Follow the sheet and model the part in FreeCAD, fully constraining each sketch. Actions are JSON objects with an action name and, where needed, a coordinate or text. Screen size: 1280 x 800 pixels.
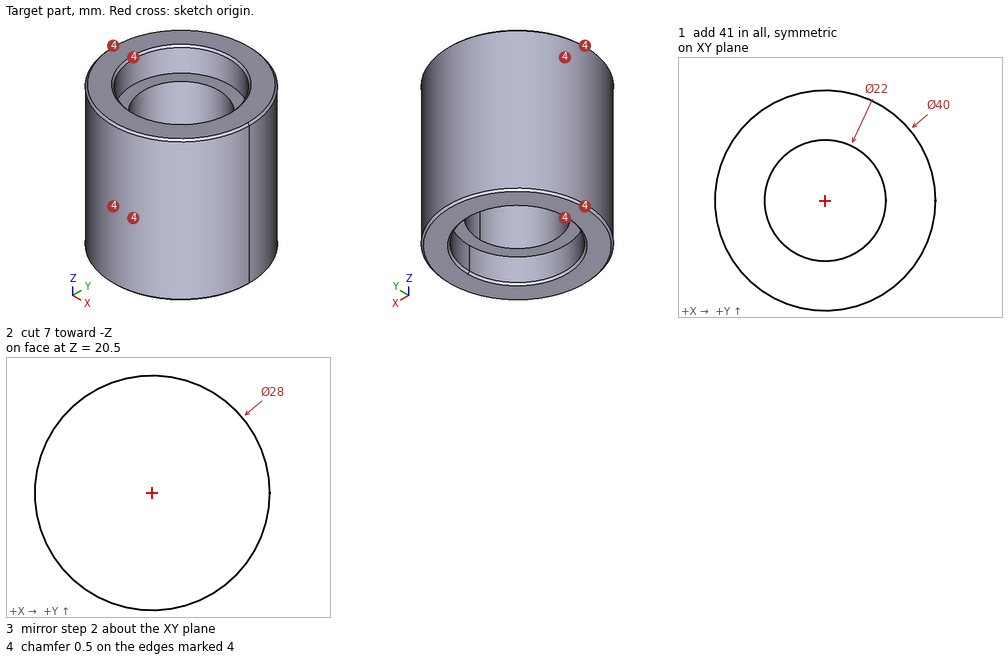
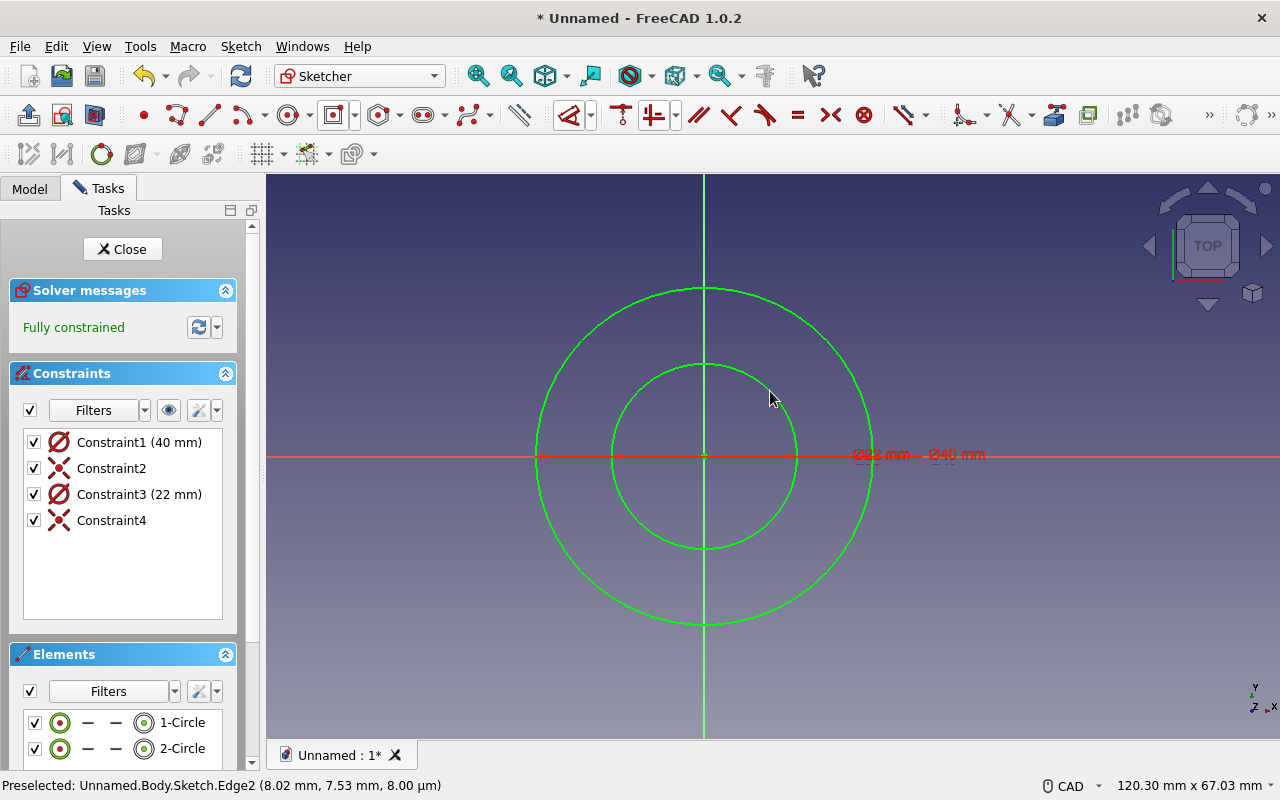
{"action": "left_click", "coordinate": [123, 249]}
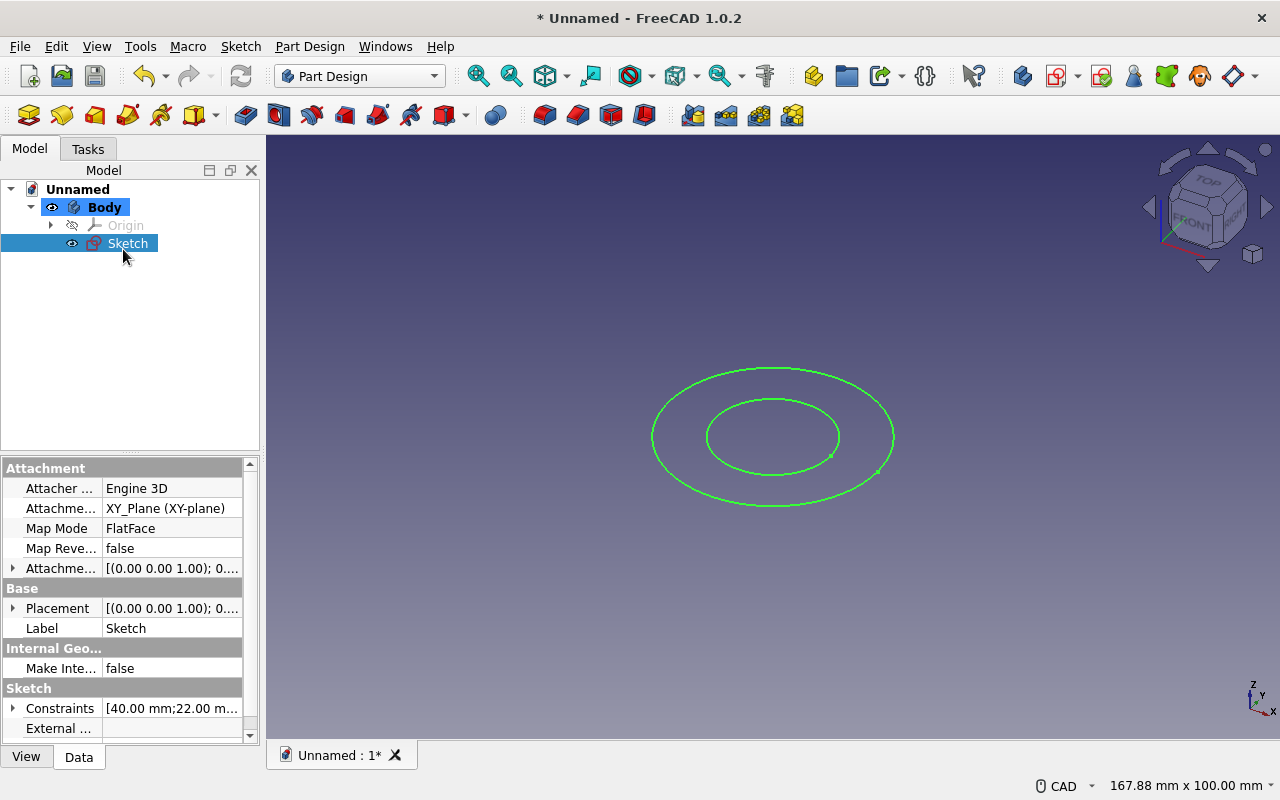
{"action": "left_click", "coordinate": [29, 116]}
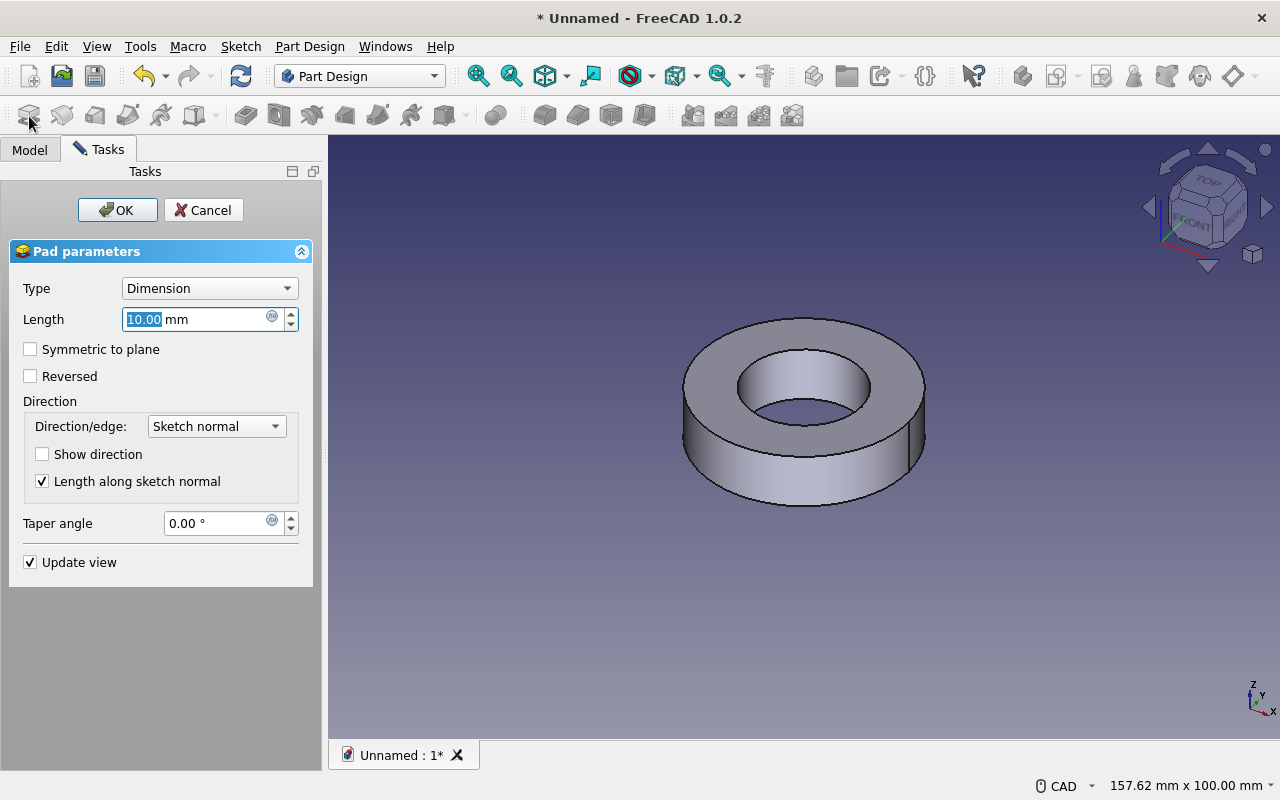
{"action": "type", "text": "41"}
{"action": "key", "text": "Tab"}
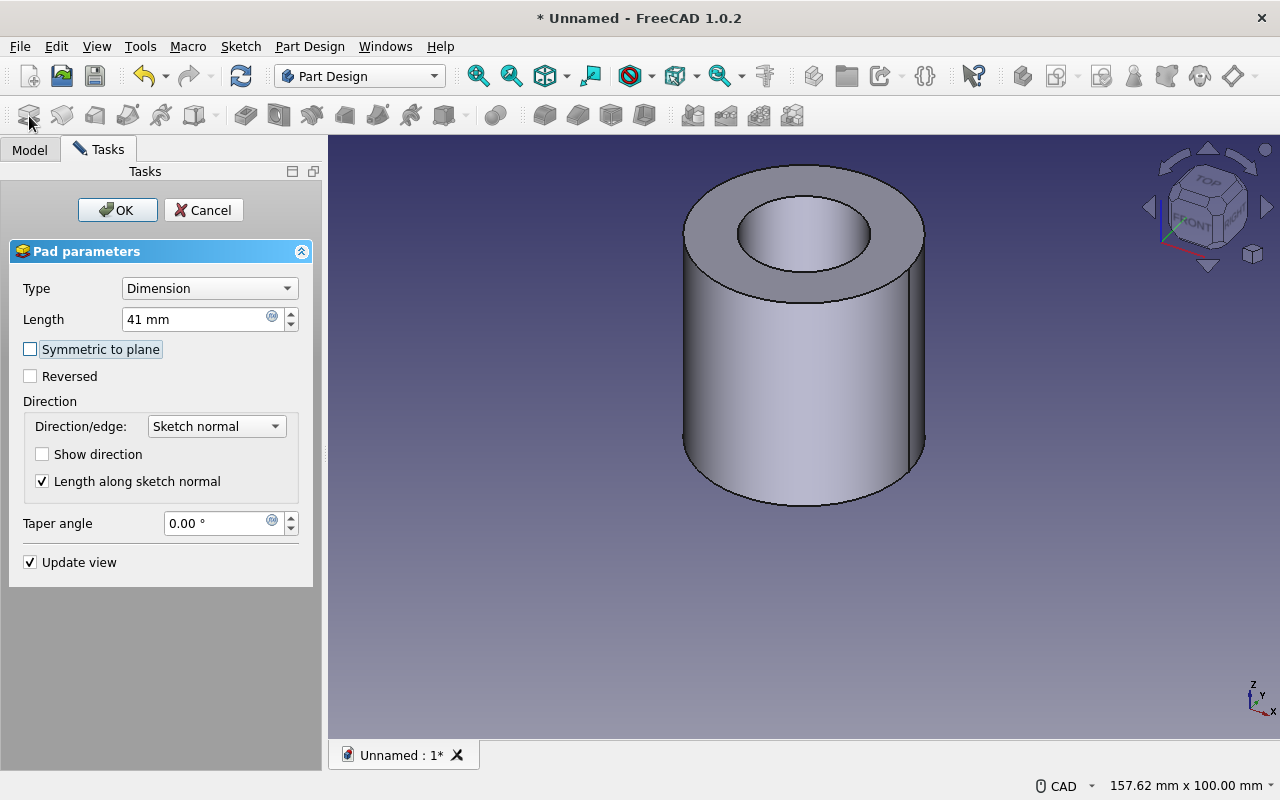
{"action": "left_click", "coordinate": [31, 349]}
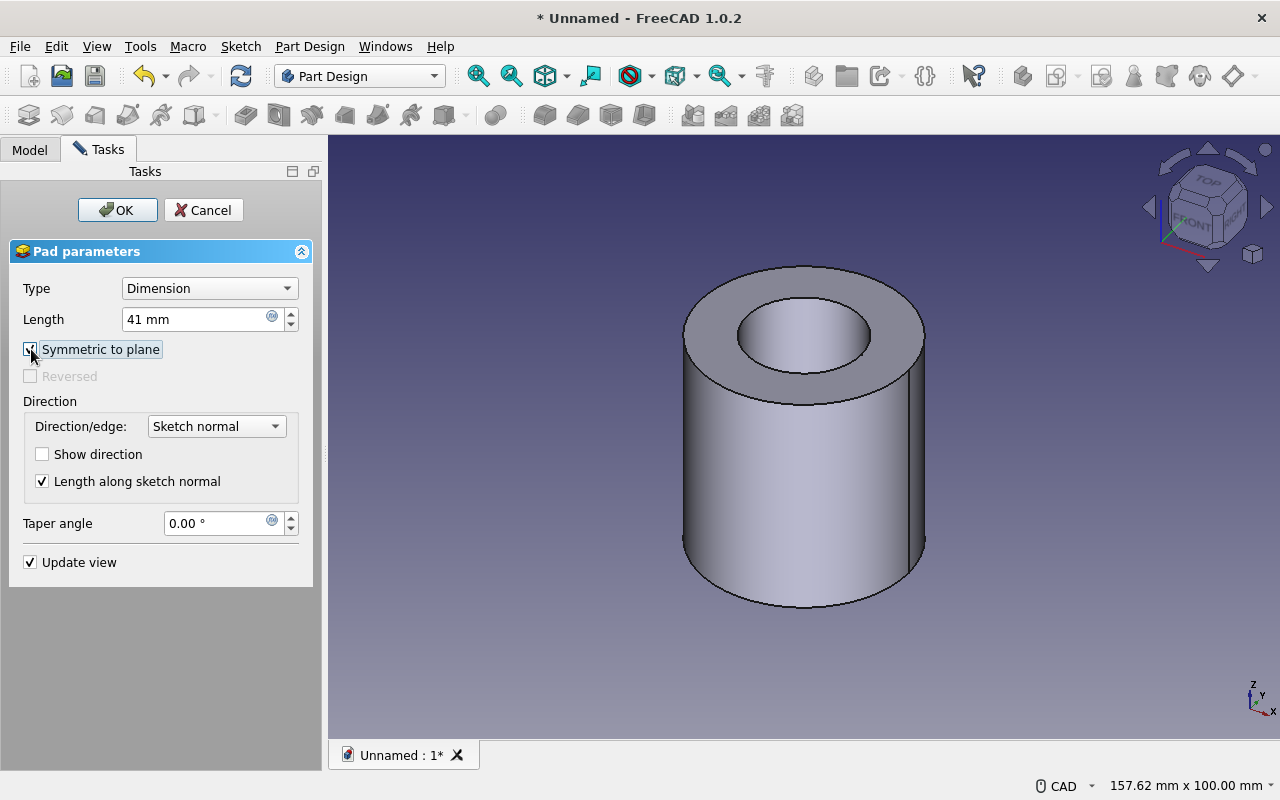
{"action": "left_click", "coordinate": [118, 210]}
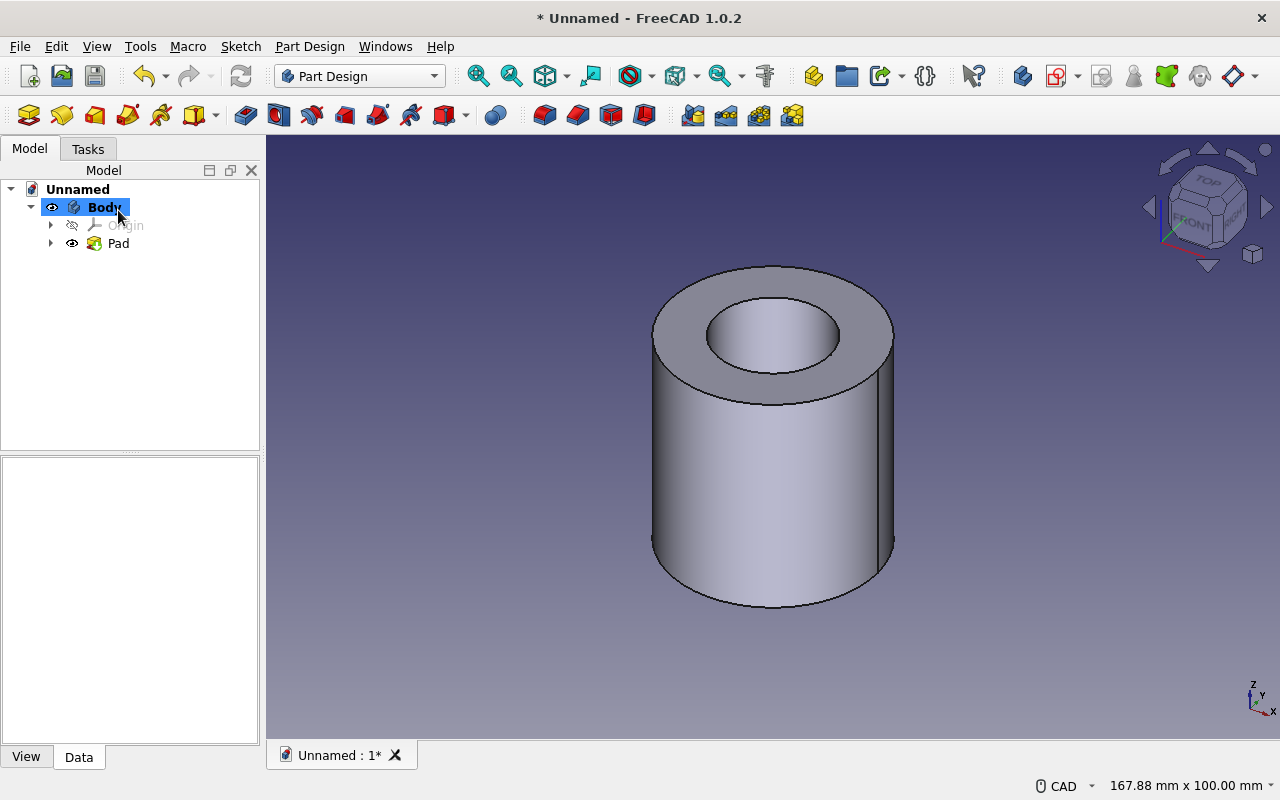
{"action": "left_click", "coordinate": [867, 320]}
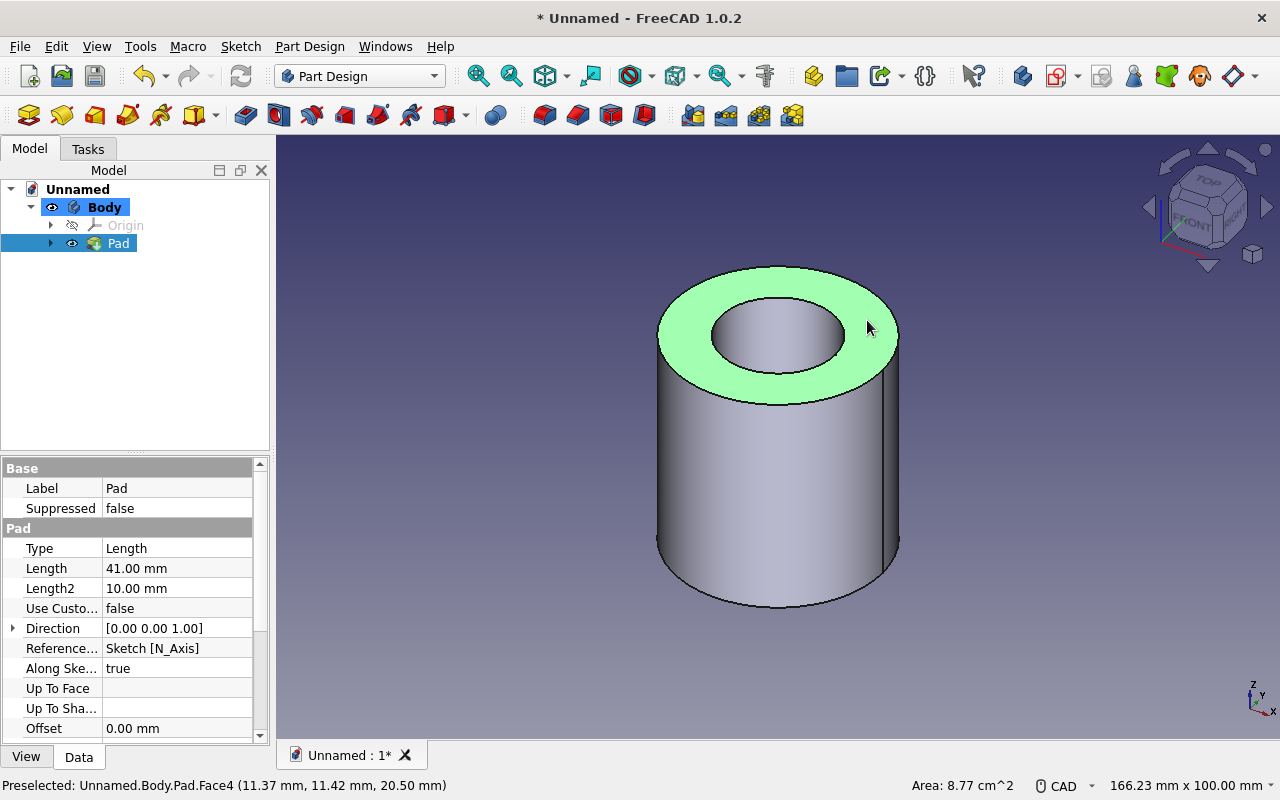
{"action": "left_click", "coordinate": [1056, 76]}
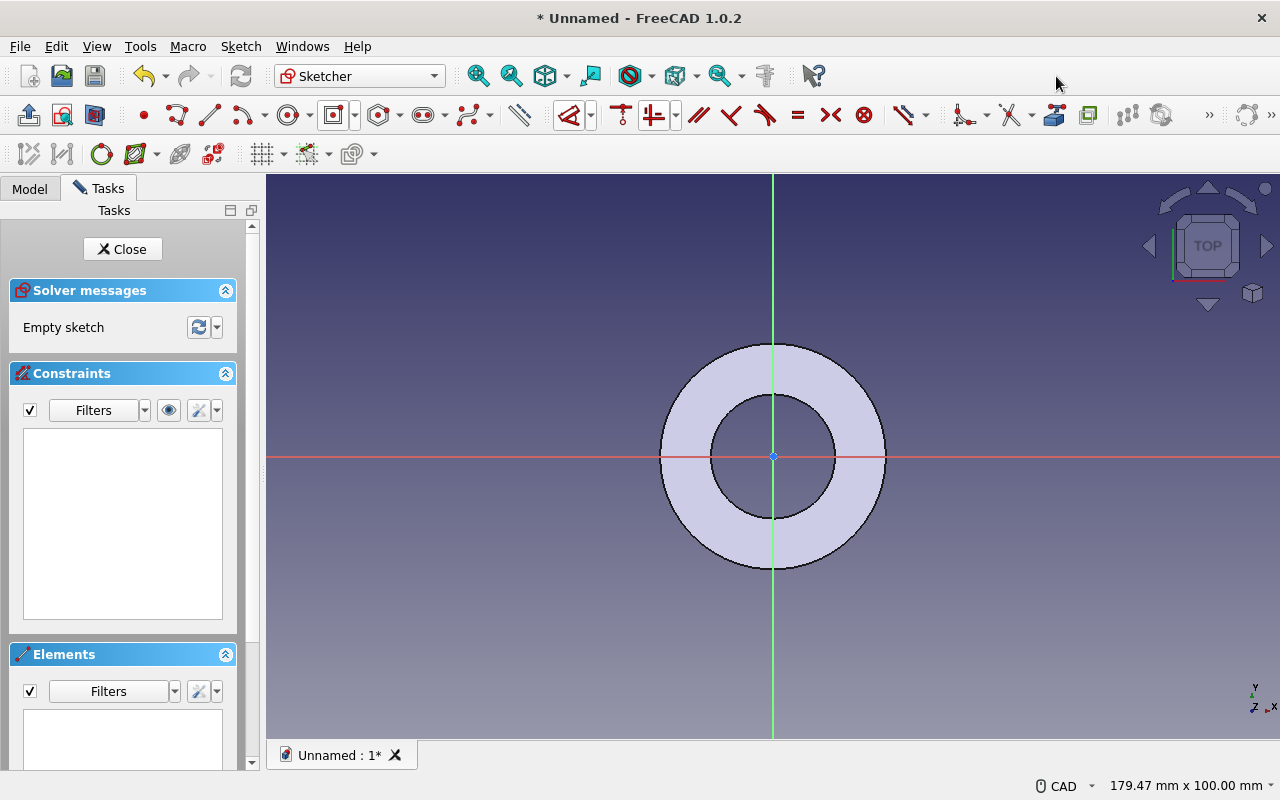
{"action": "scroll", "coordinate": [829, 456], "scroll_direction": "up", "scroll_amount": 4}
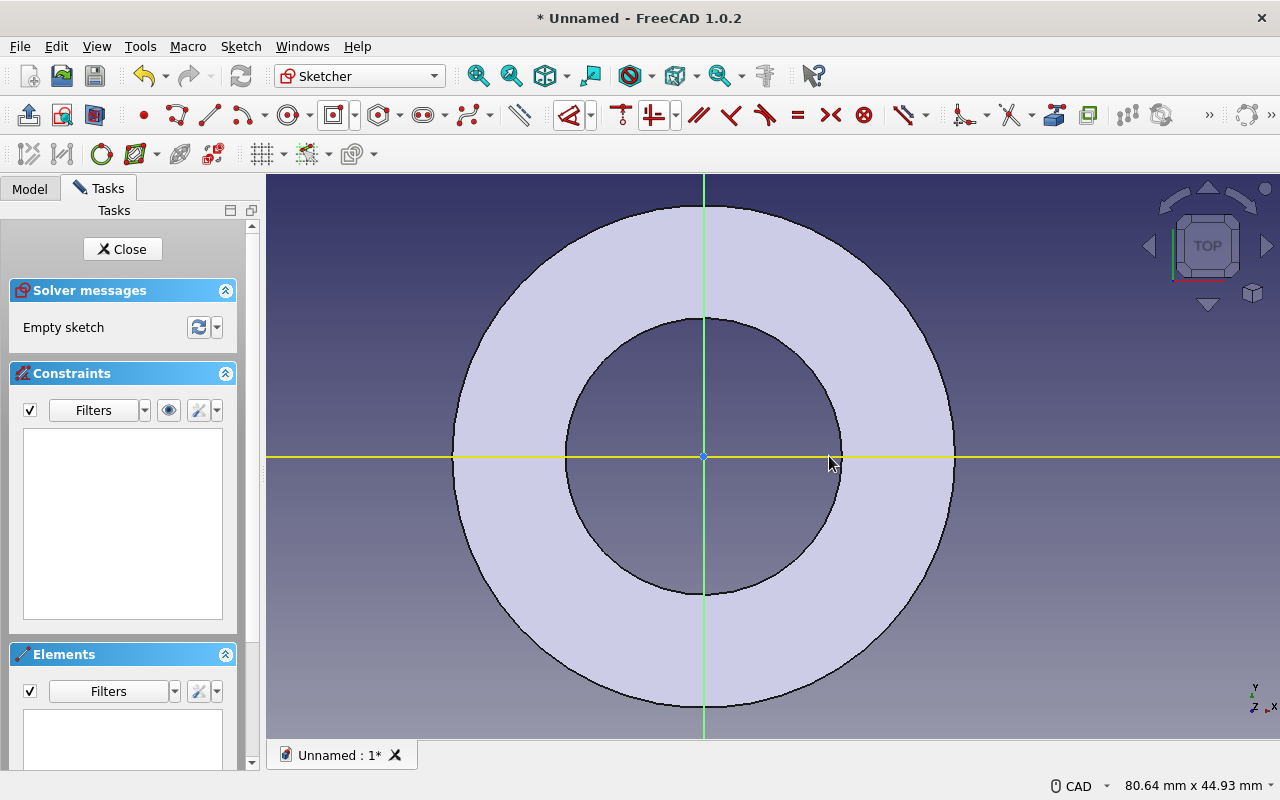
{"action": "left_click", "coordinate": [288, 116]}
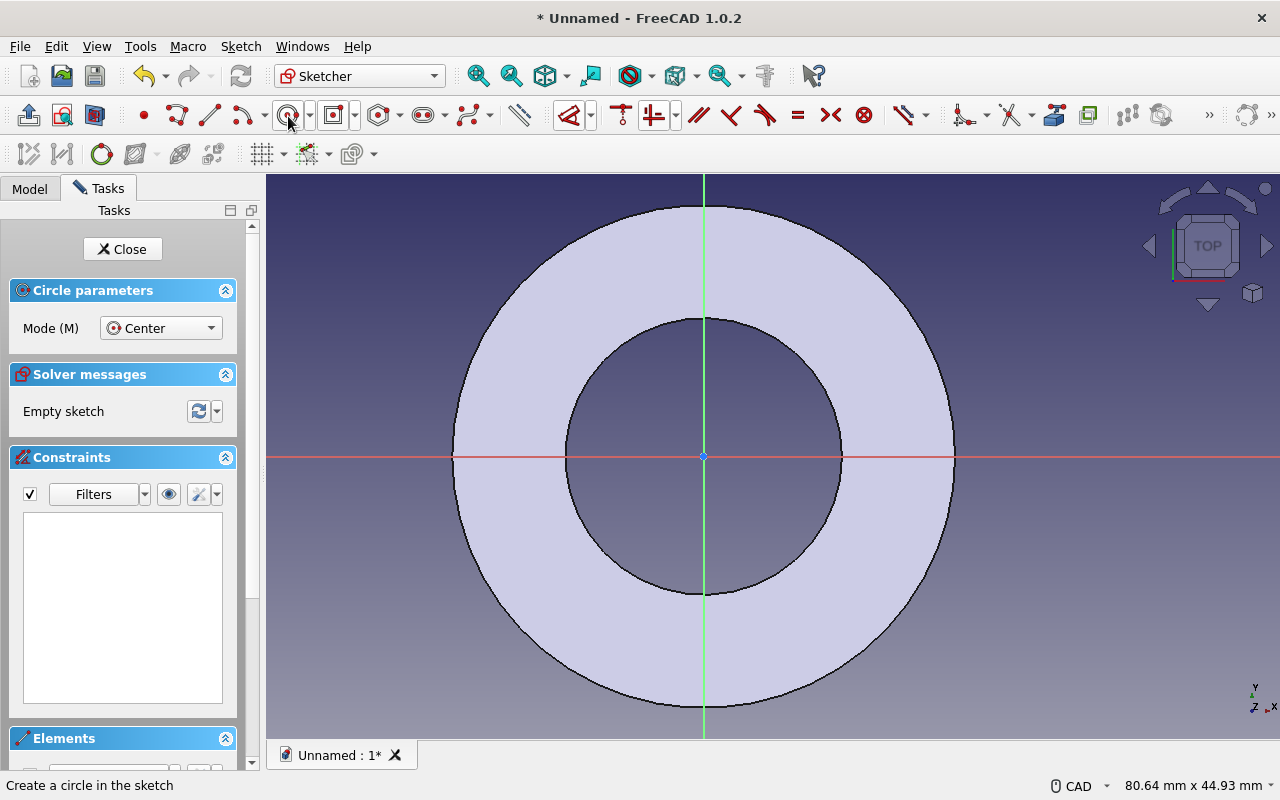
{"action": "left_click", "coordinate": [704, 456]}
{"action": "mouse_move", "coordinate": [828, 332]}